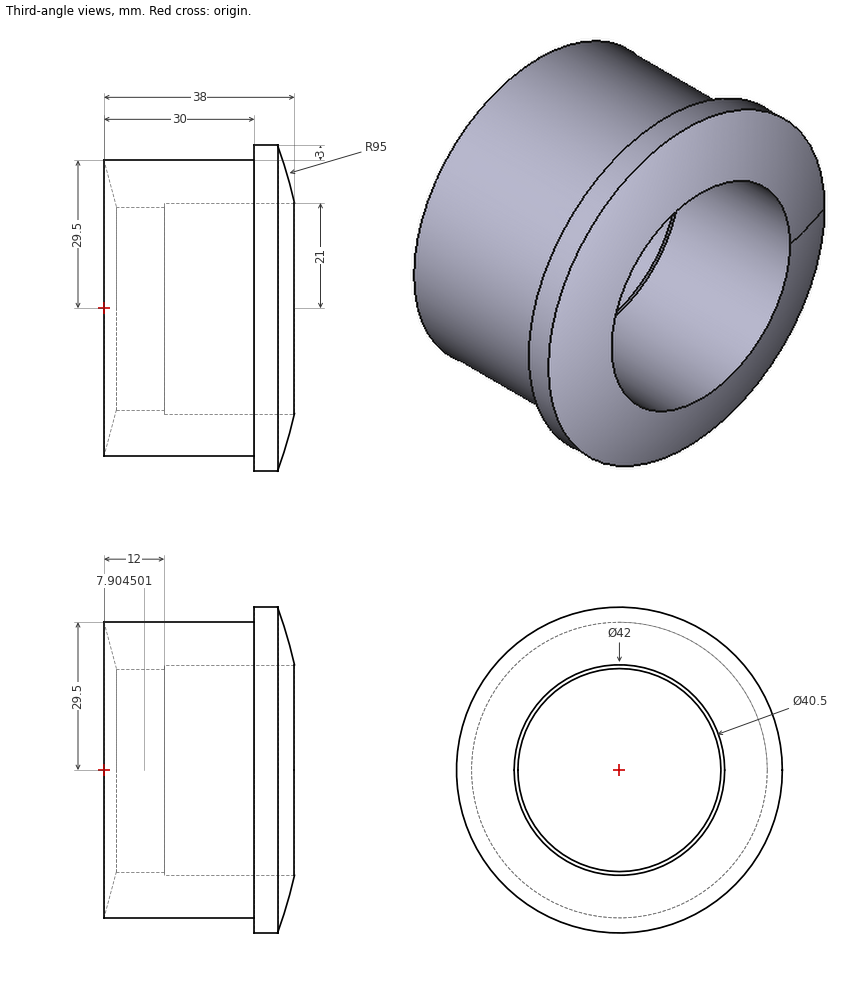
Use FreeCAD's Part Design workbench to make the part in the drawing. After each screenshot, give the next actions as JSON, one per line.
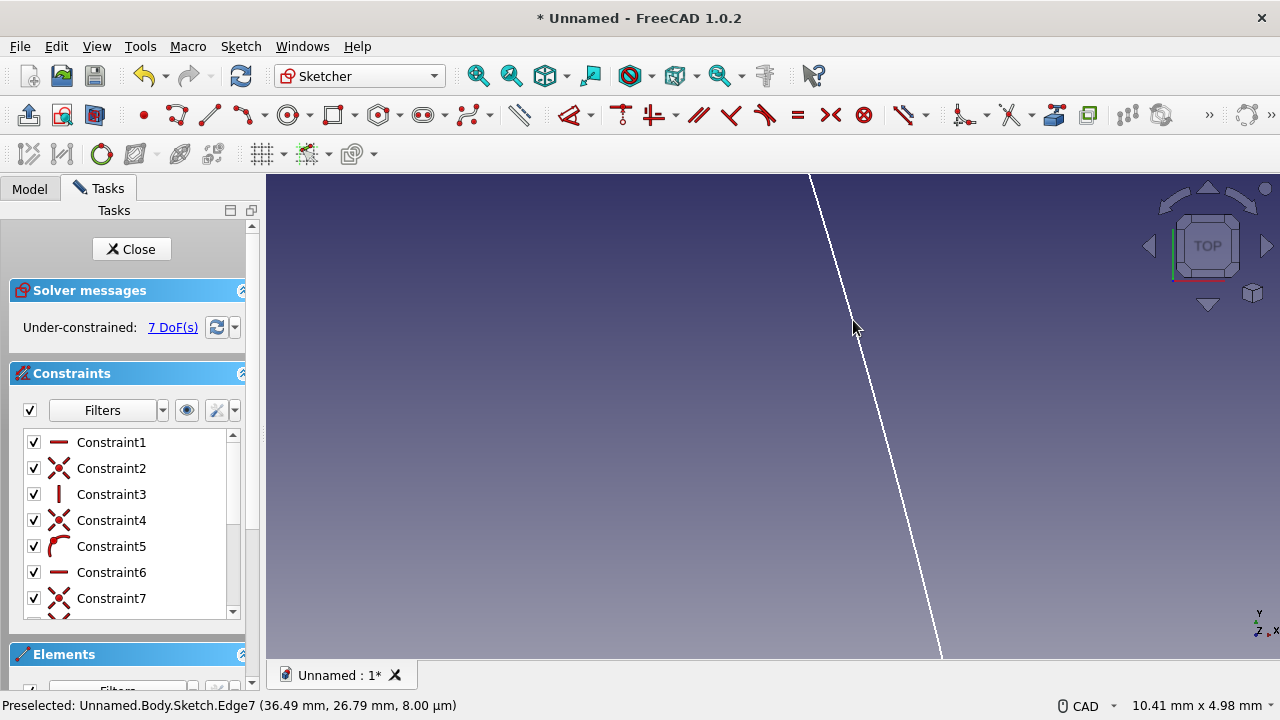
{"action": "scroll", "coordinate": [860, 324], "scroll_direction": "down", "scroll_amount": 12}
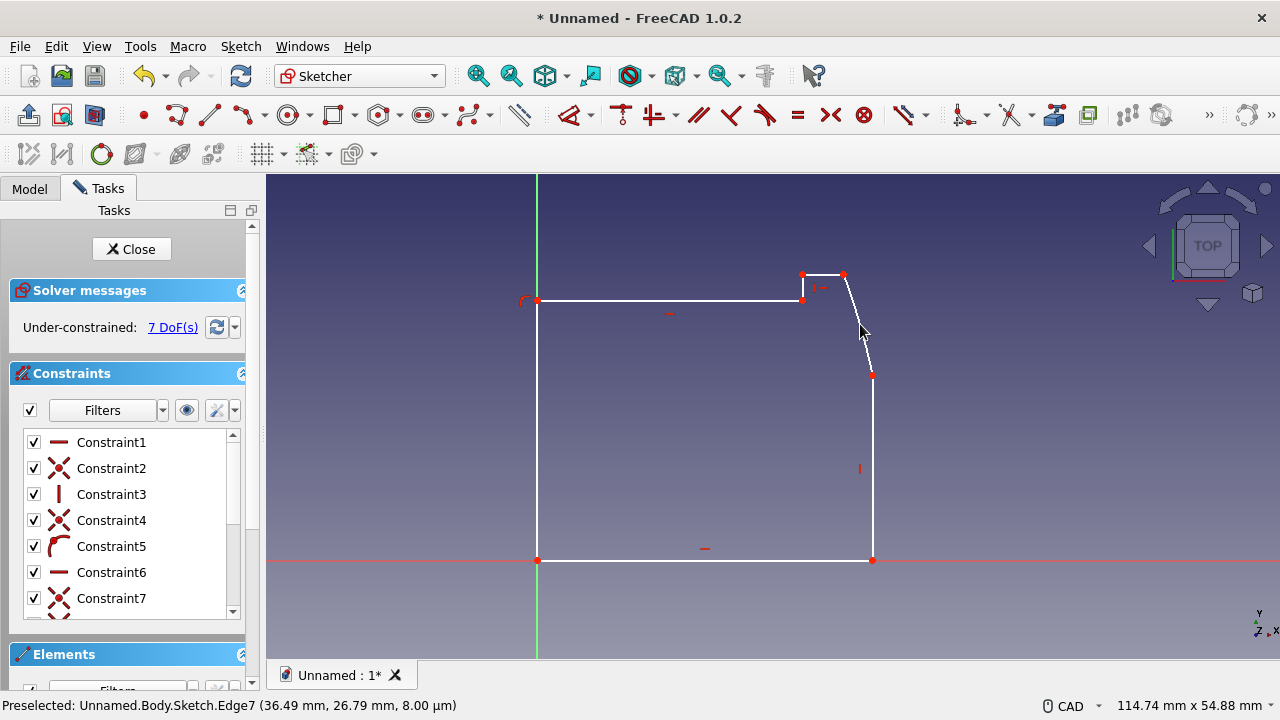
{"action": "scroll", "coordinate": [1115, 414], "scroll_direction": "down", "scroll_amount": 1}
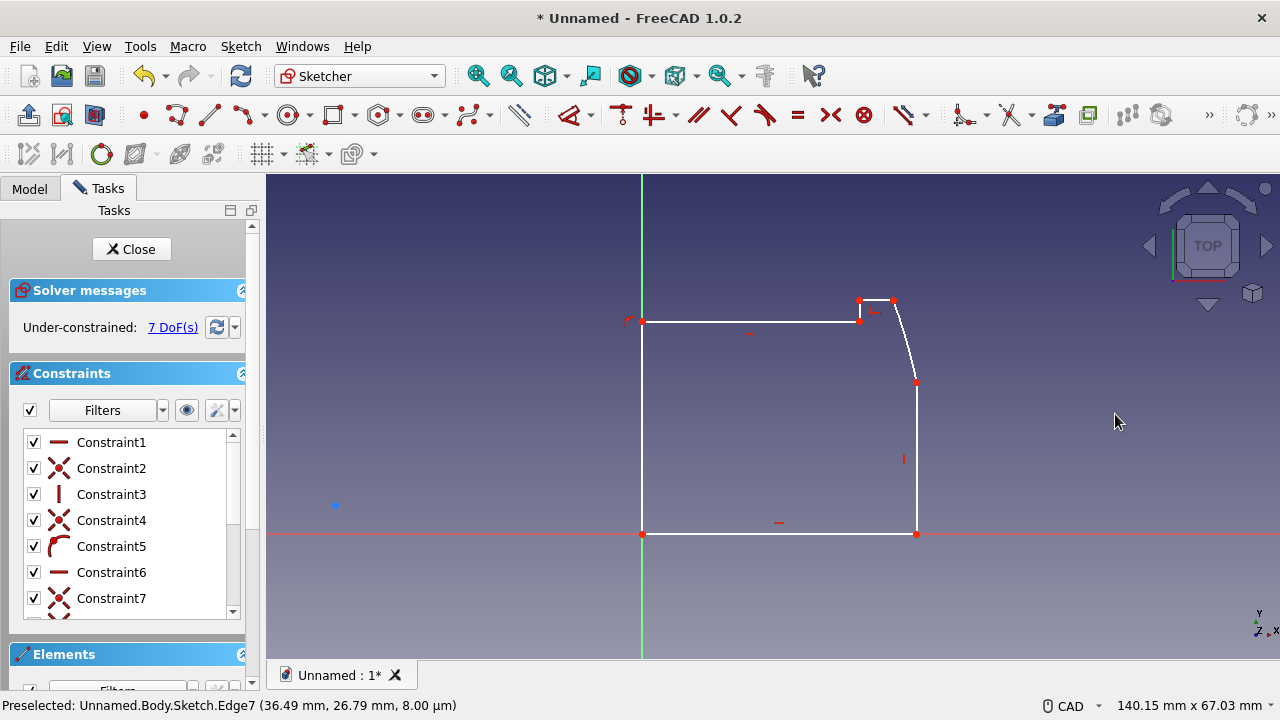
{"action": "left_click", "coordinate": [335, 505]}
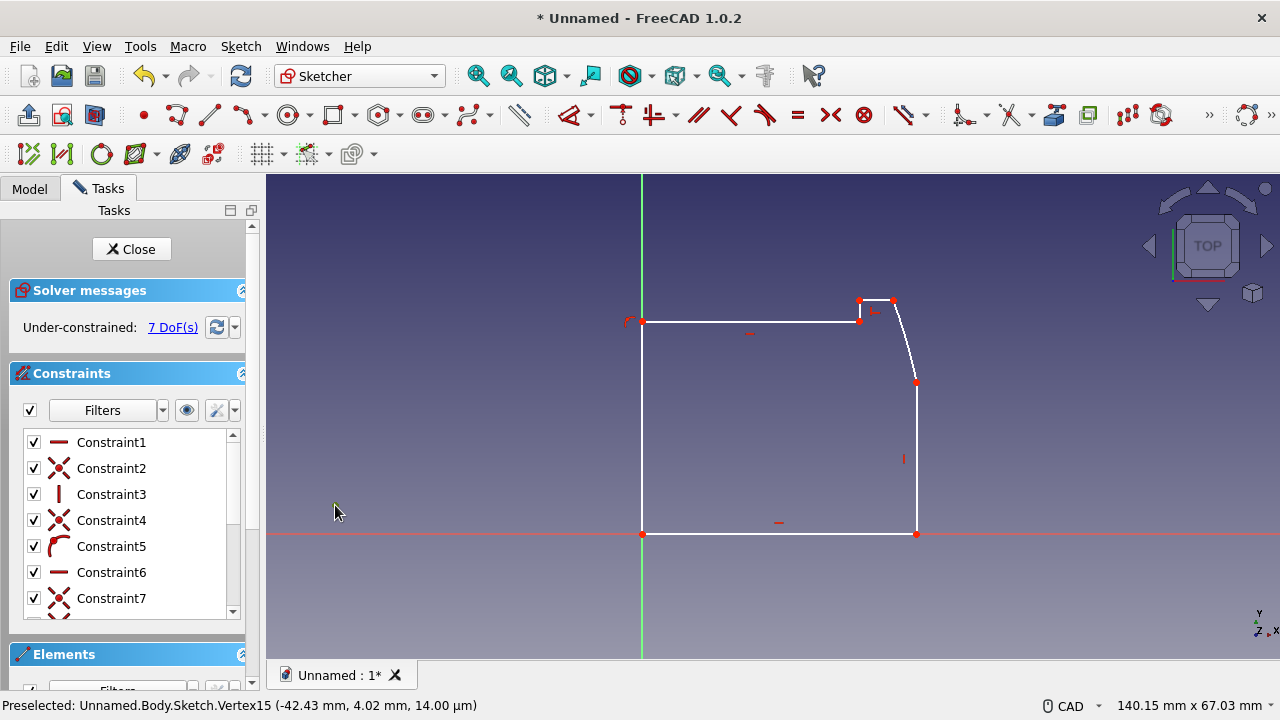
{"action": "left_click", "coordinate": [353, 534]}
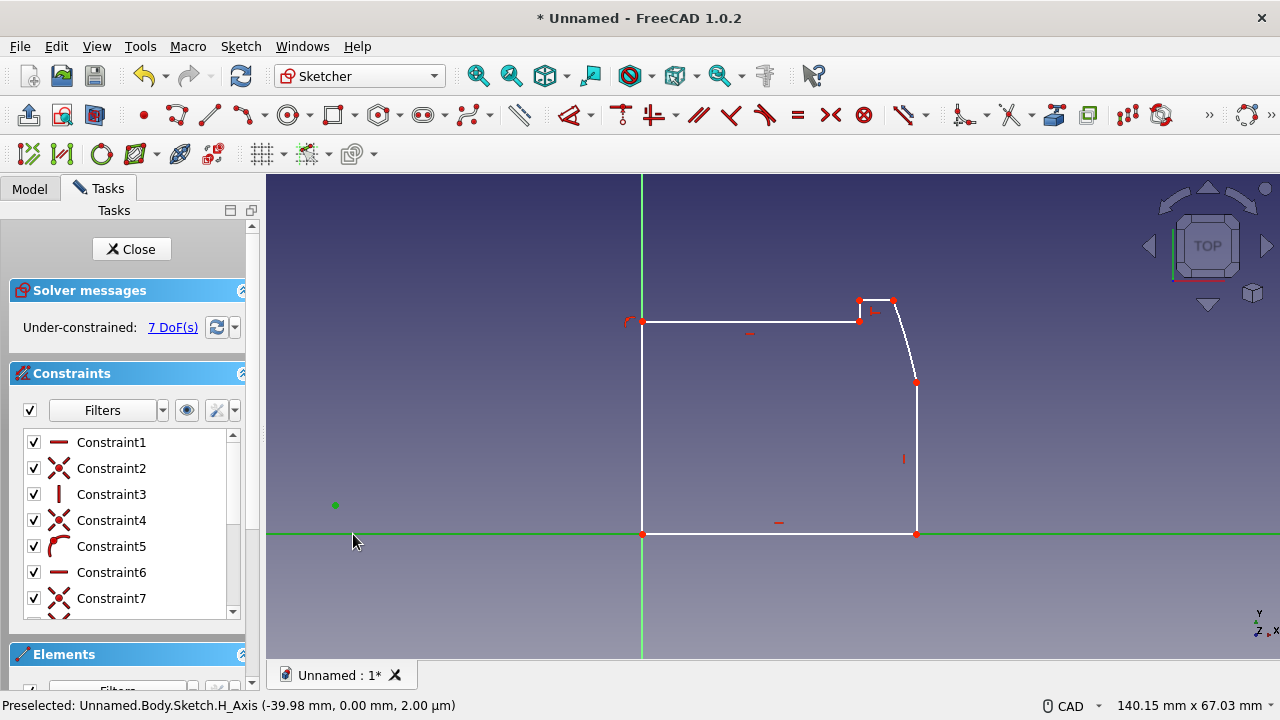
{"action": "left_click", "coordinate": [621, 116]}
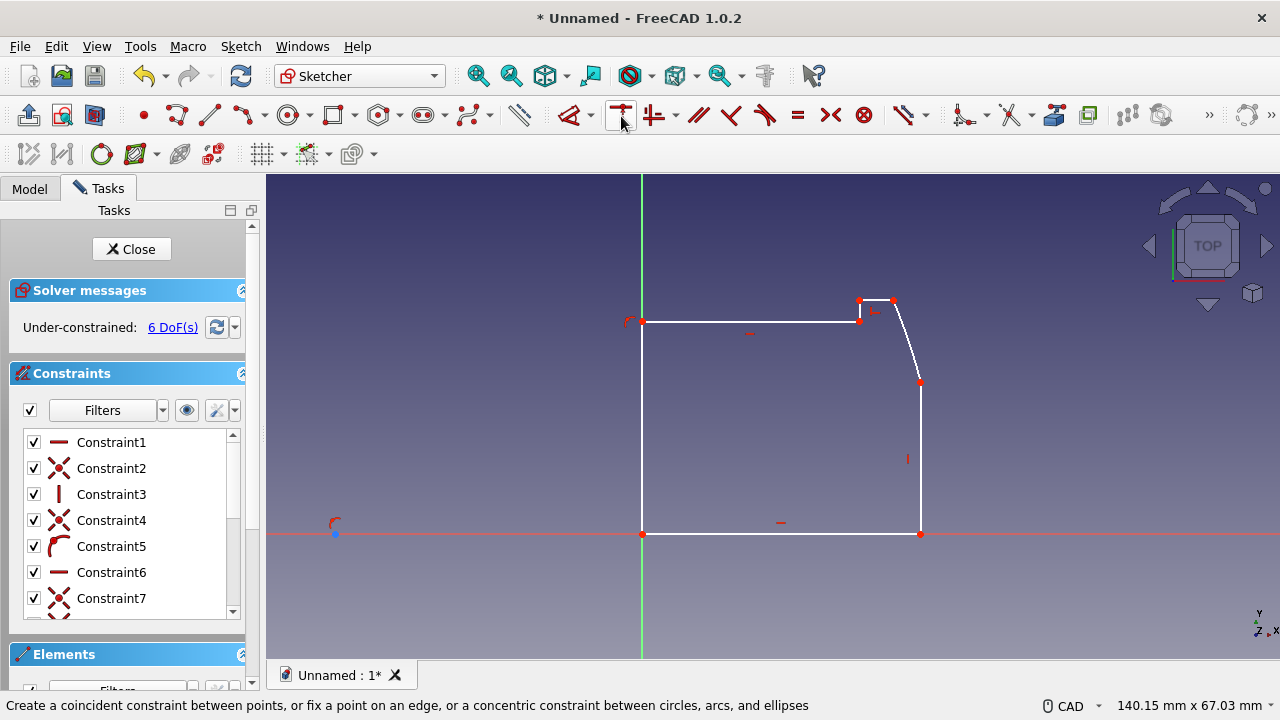
{"action": "left_click", "coordinate": [568, 116]}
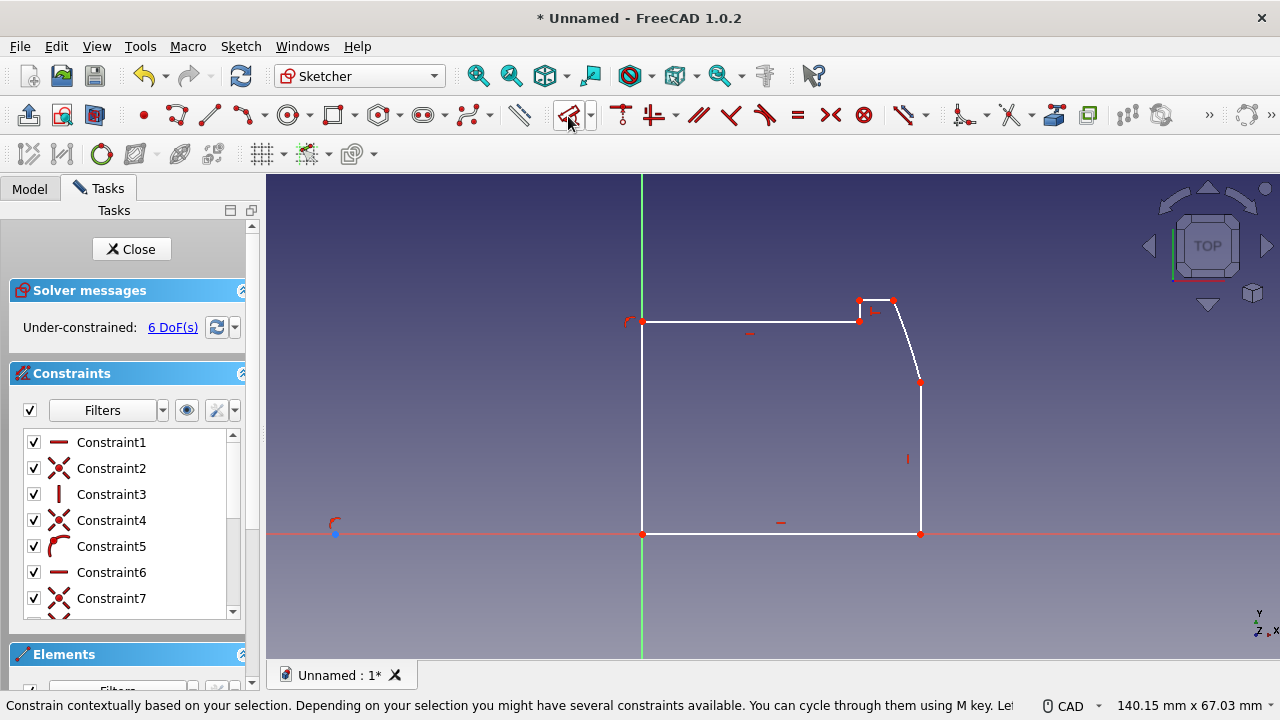
{"action": "left_click", "coordinate": [914, 358]}
{"action": "left_click", "coordinate": [945, 349]}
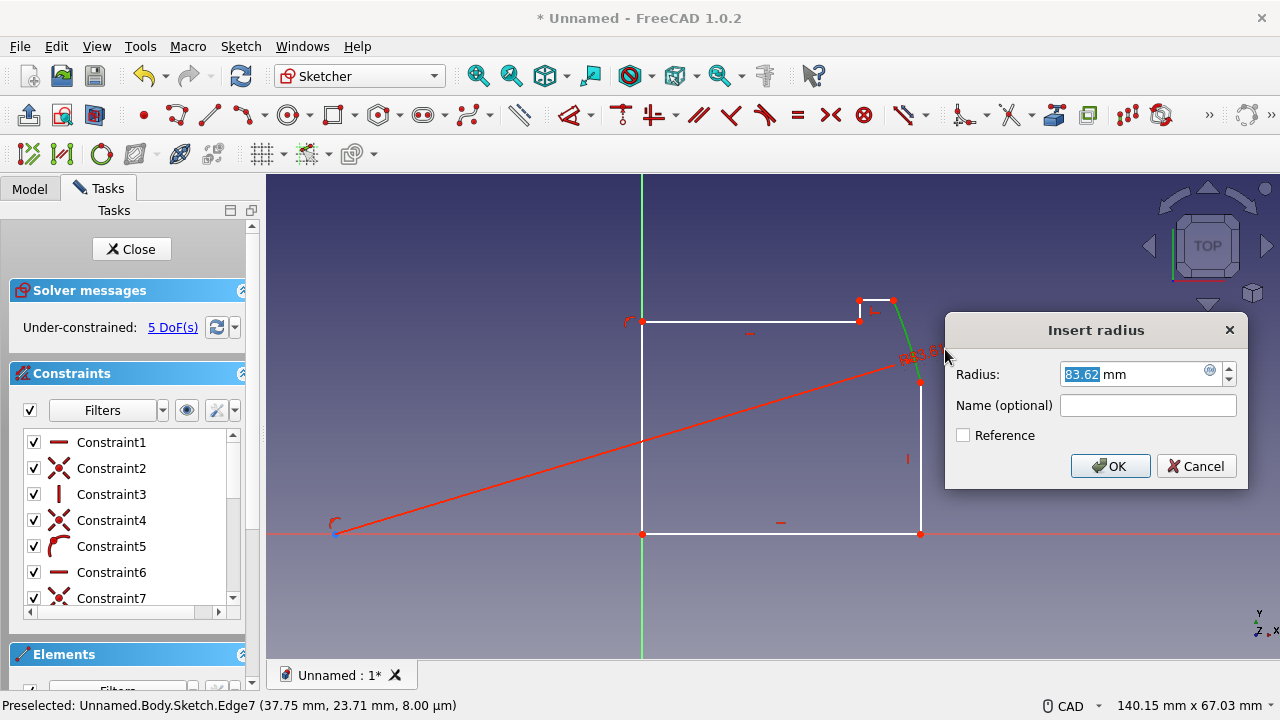
{"action": "type", "text": "95"}
{"action": "key", "text": "Return"}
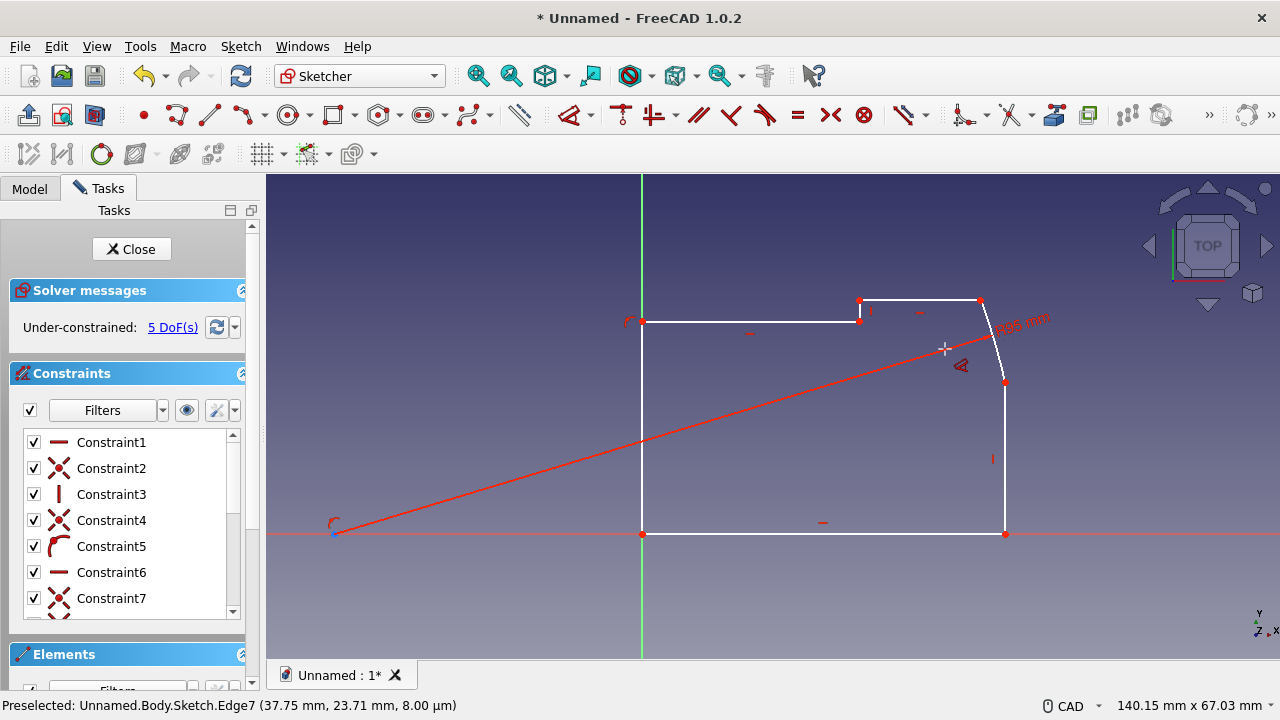
{"action": "scroll", "coordinate": [860, 311], "scroll_direction": "up", "scroll_amount": 4}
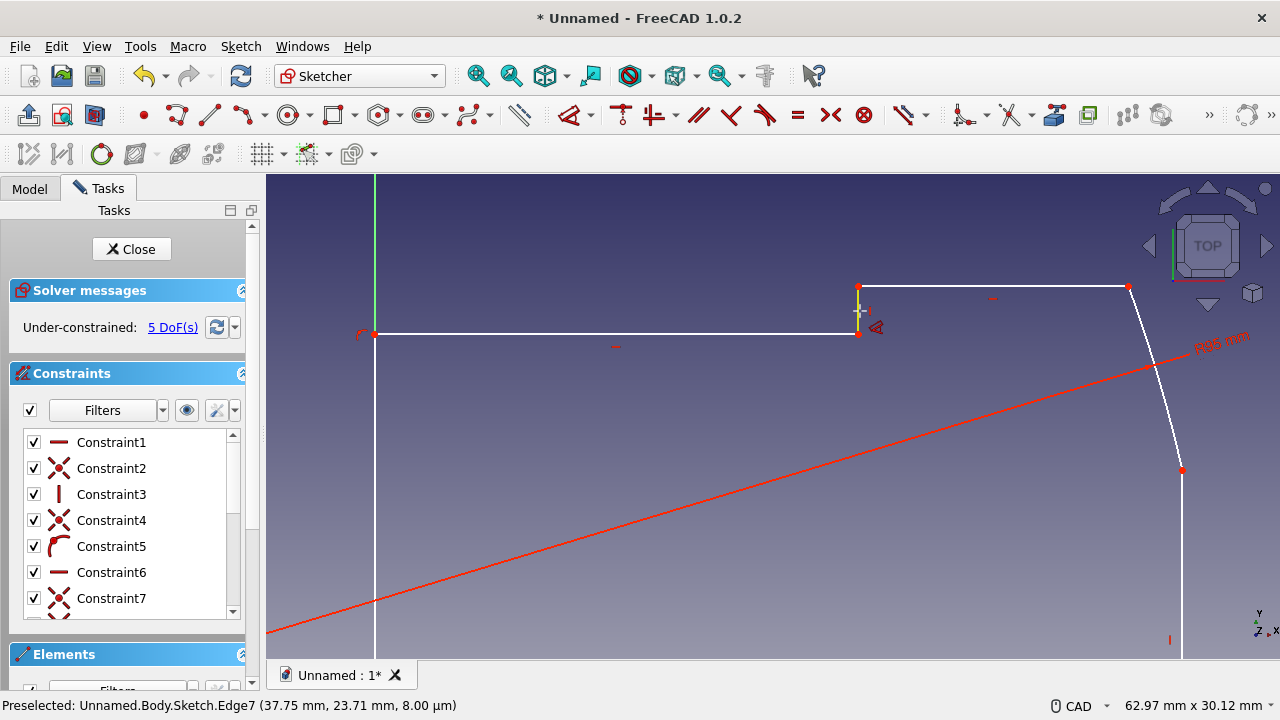
{"action": "left_click", "coordinate": [858, 310]}
{"action": "left_click", "coordinate": [892, 310]}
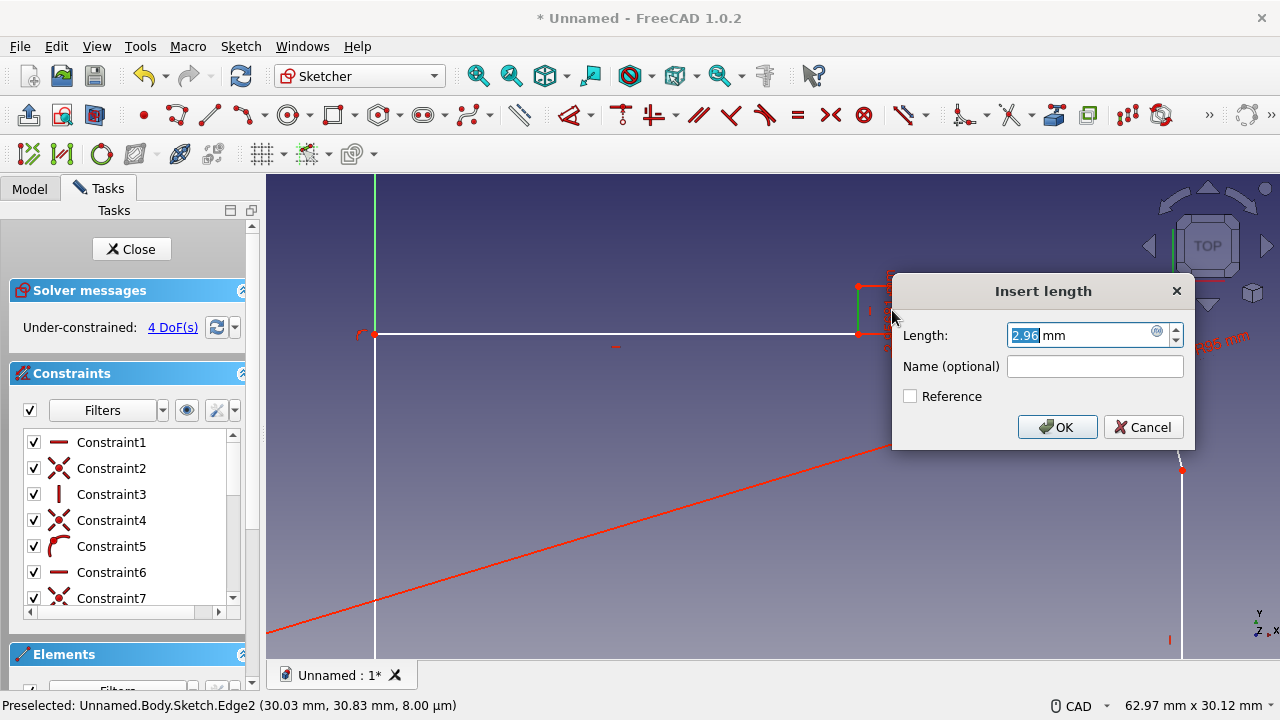
{"action": "type", "text": "3"}
{"action": "key", "text": "Return"}